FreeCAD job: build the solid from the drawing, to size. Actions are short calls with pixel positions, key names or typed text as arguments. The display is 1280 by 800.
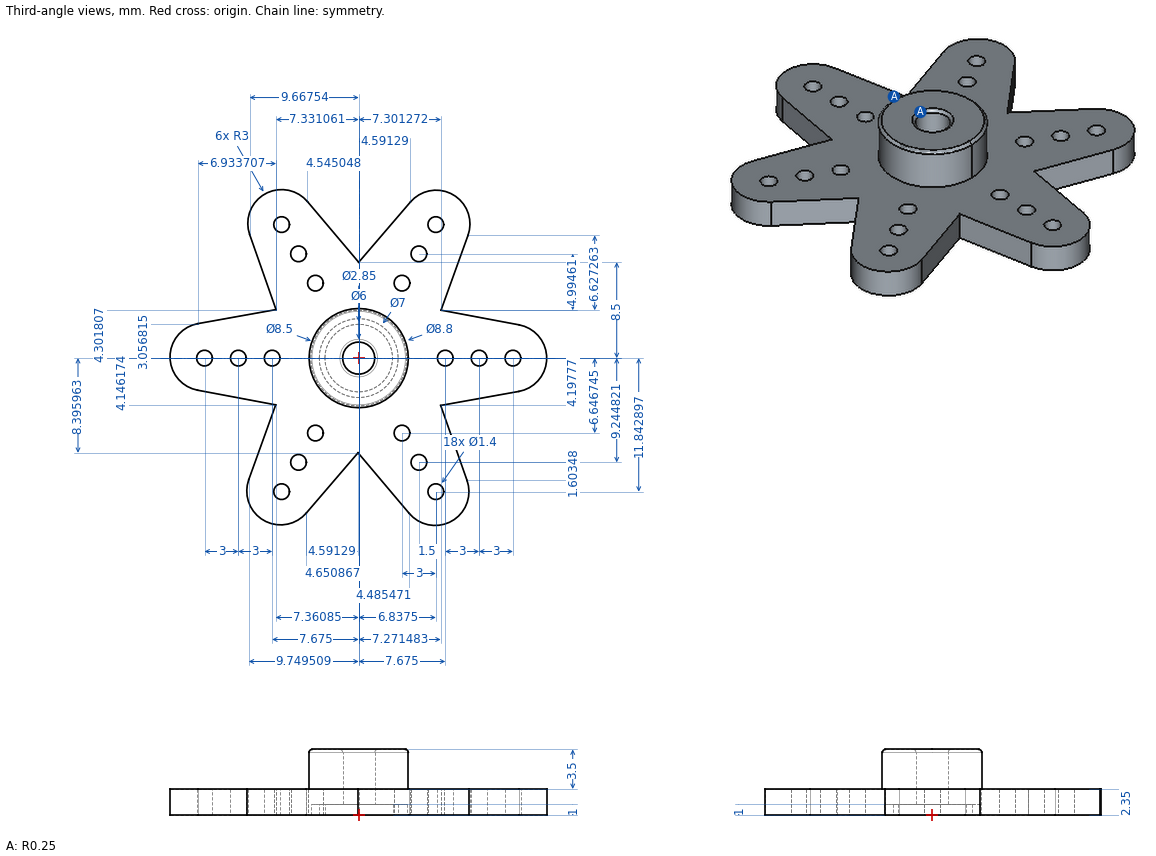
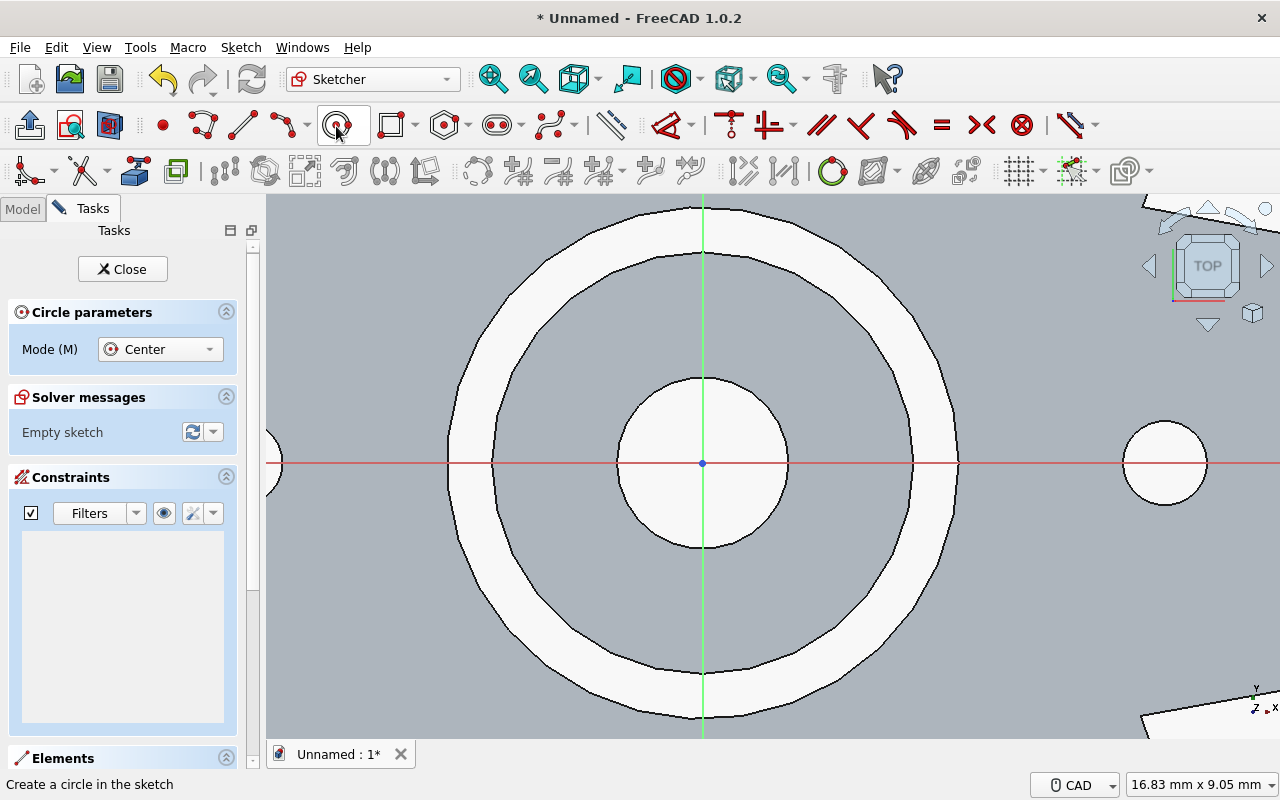
click(703, 463)
click(831, 335)
key(Escape)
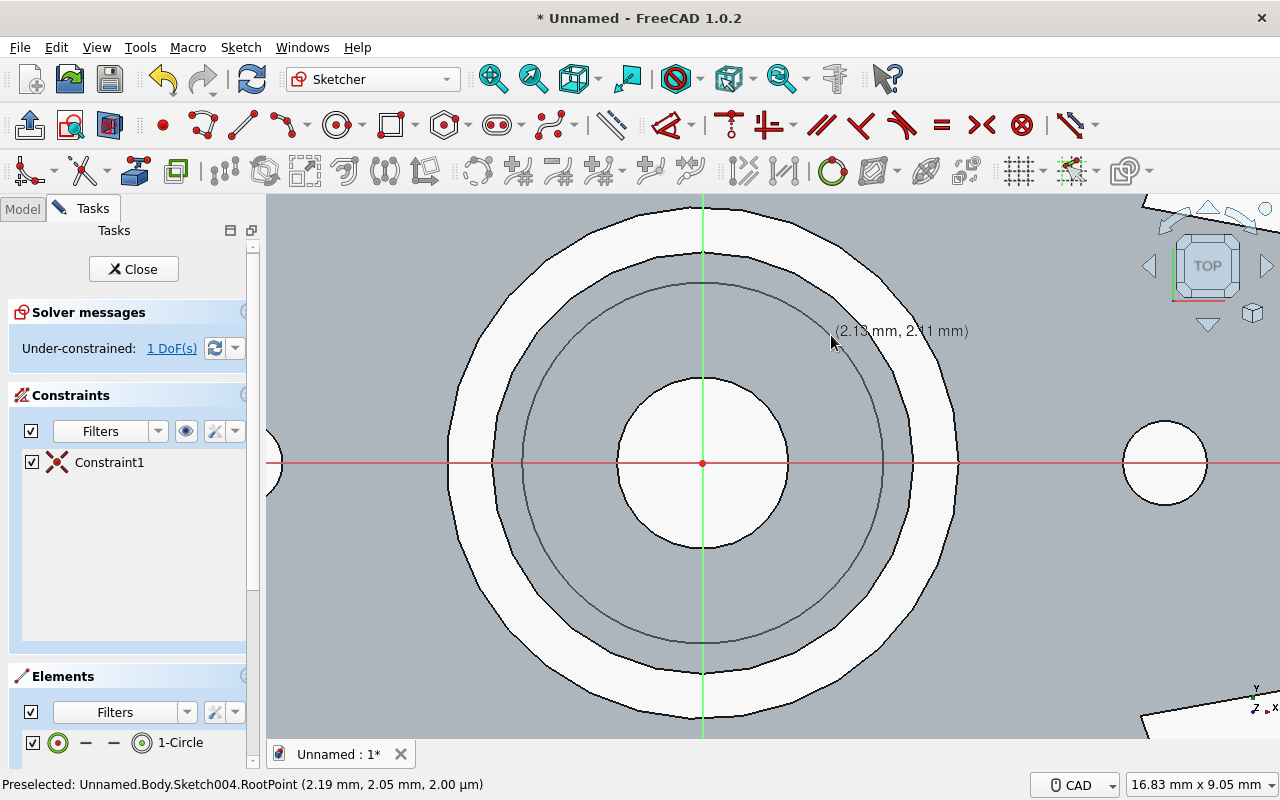
click(666, 126)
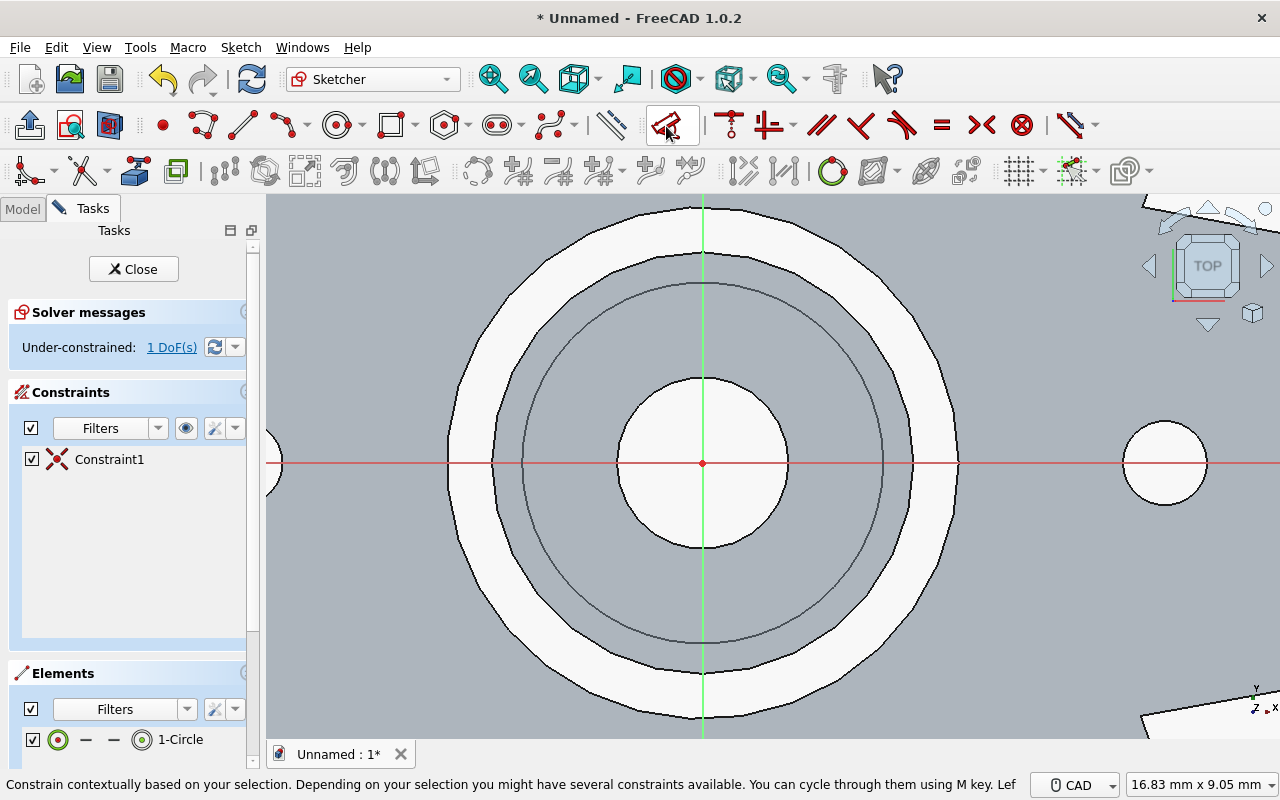
click(830, 335)
click(853, 312)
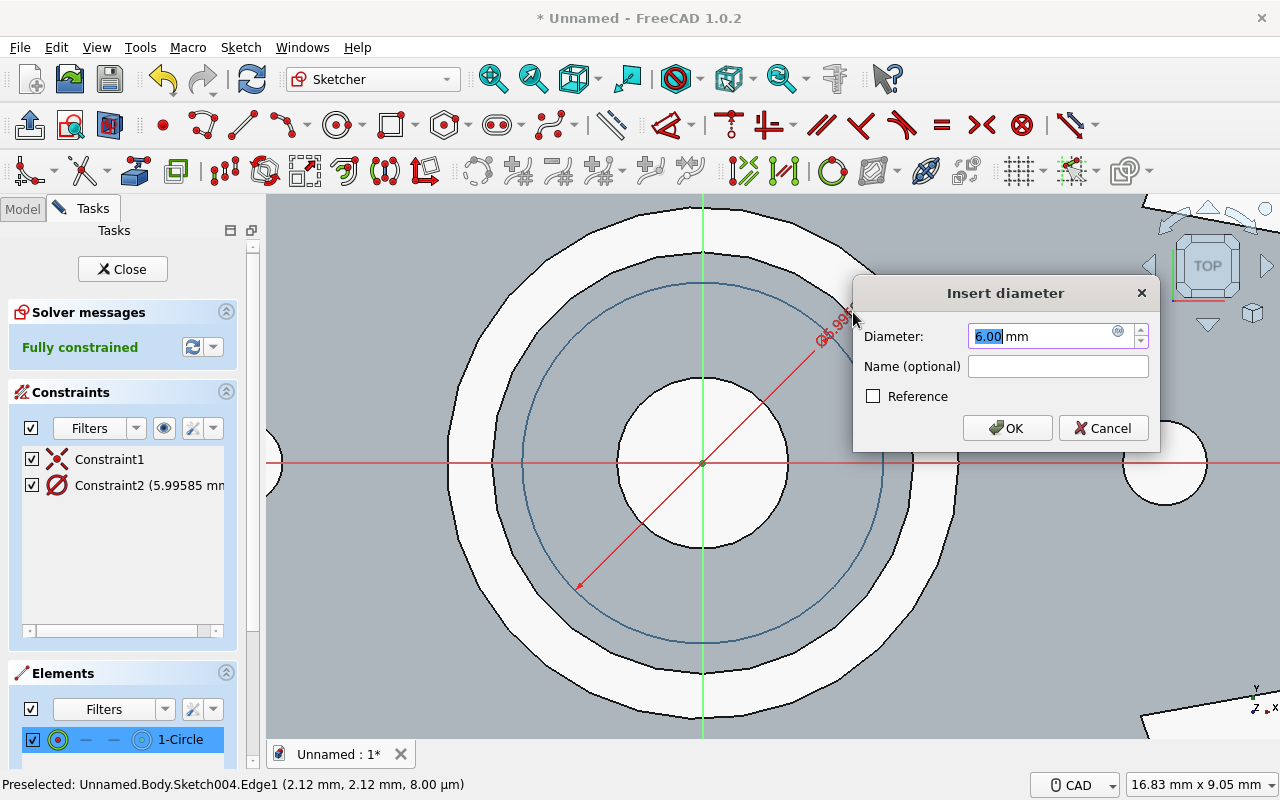
text(6)
key(Return)
key(Escape)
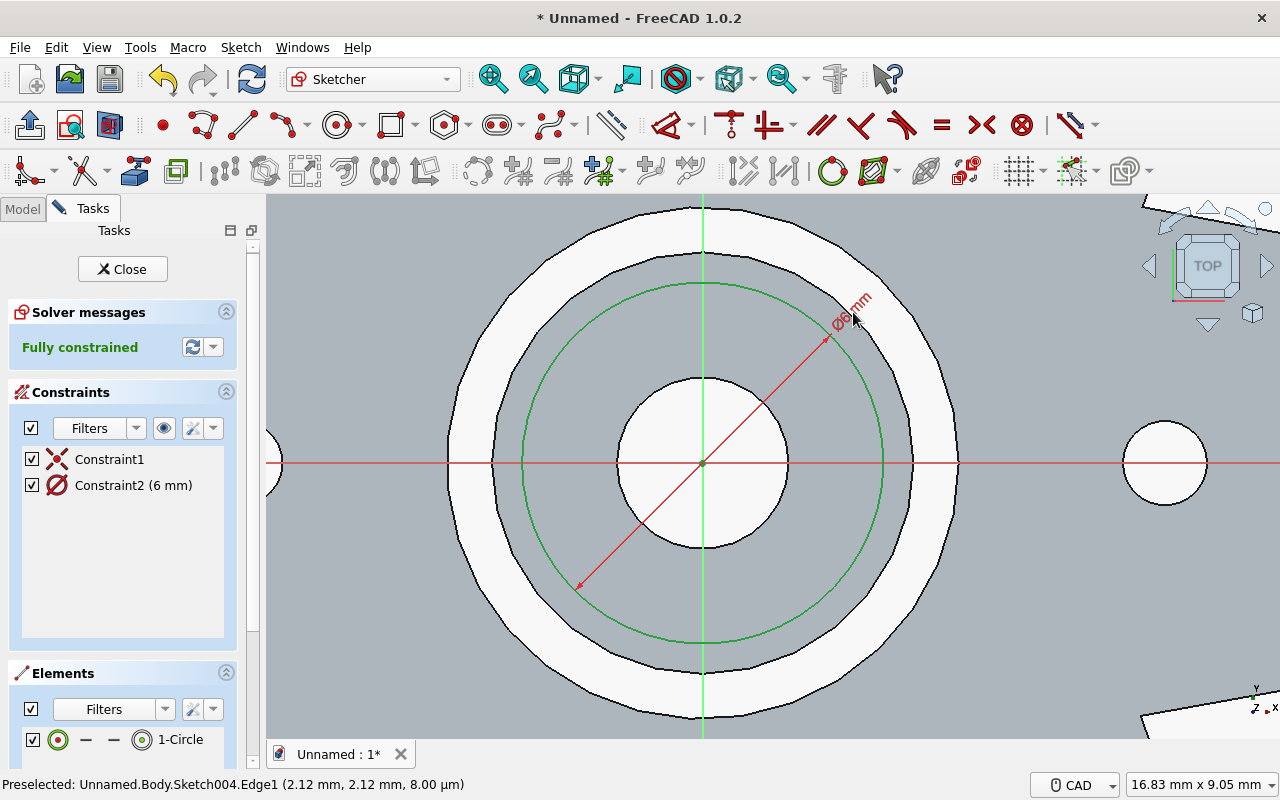
click(123, 269)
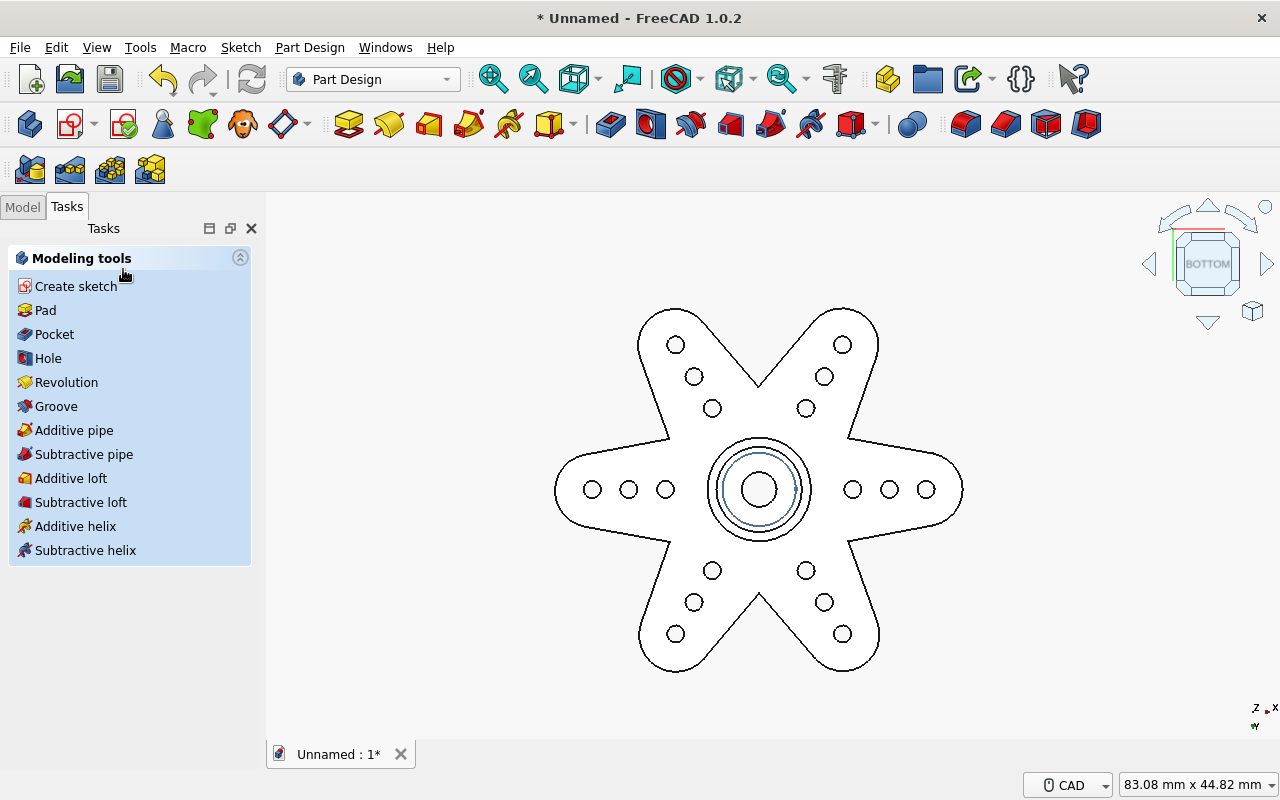
click(612, 124)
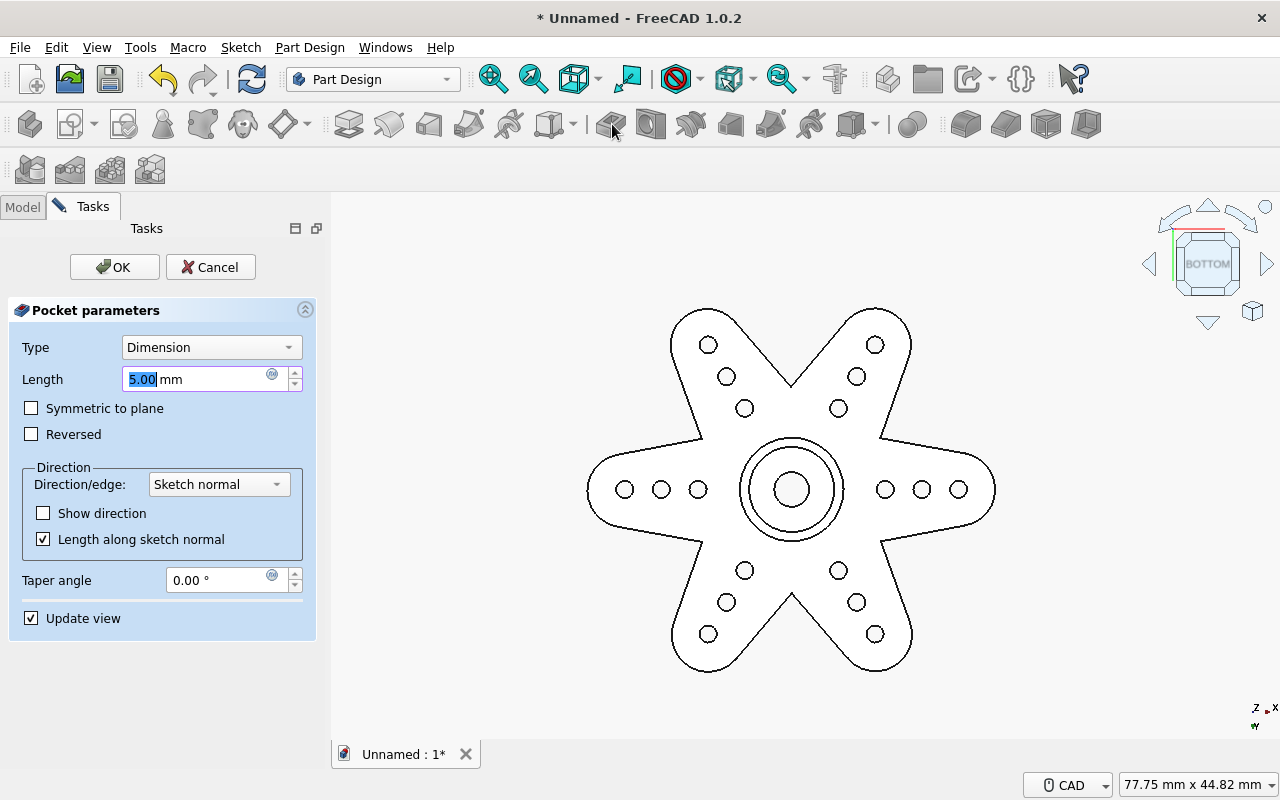
text(1)
key(Tab)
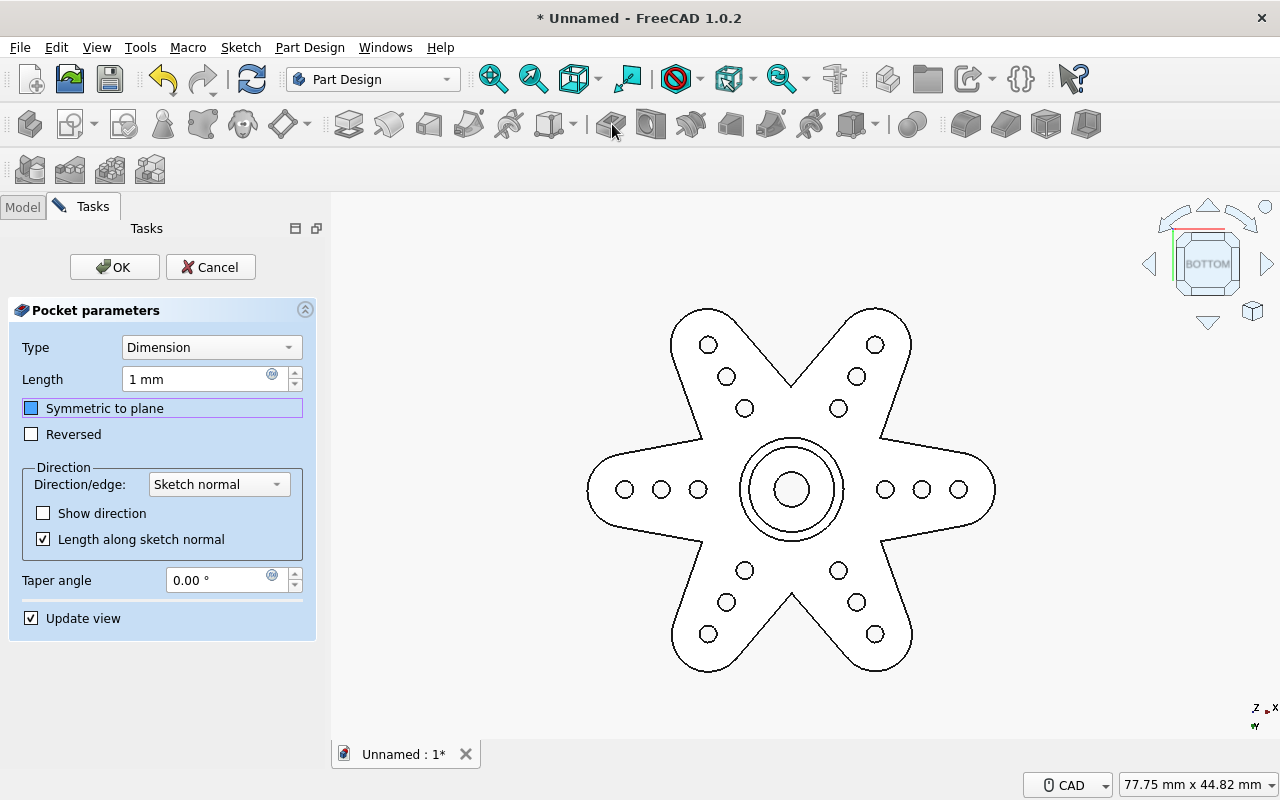
click(30, 434)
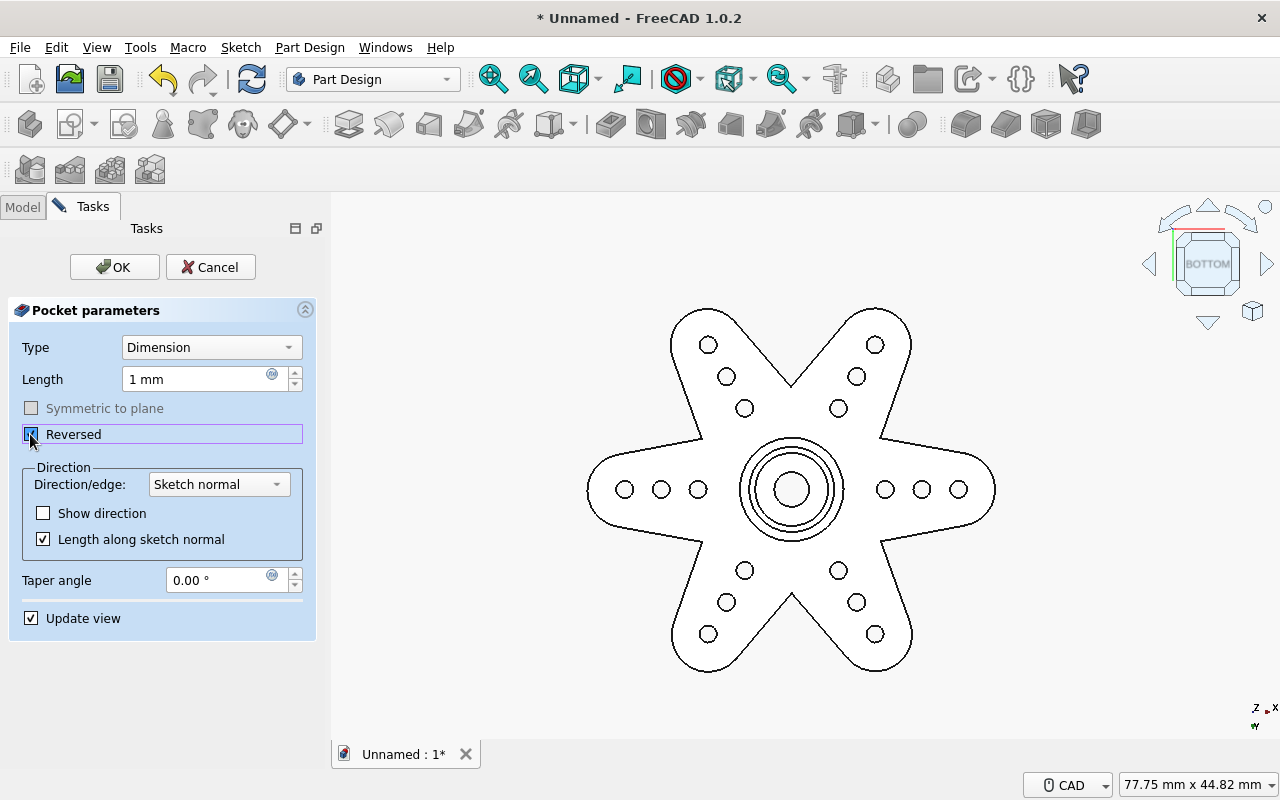
click(115, 267)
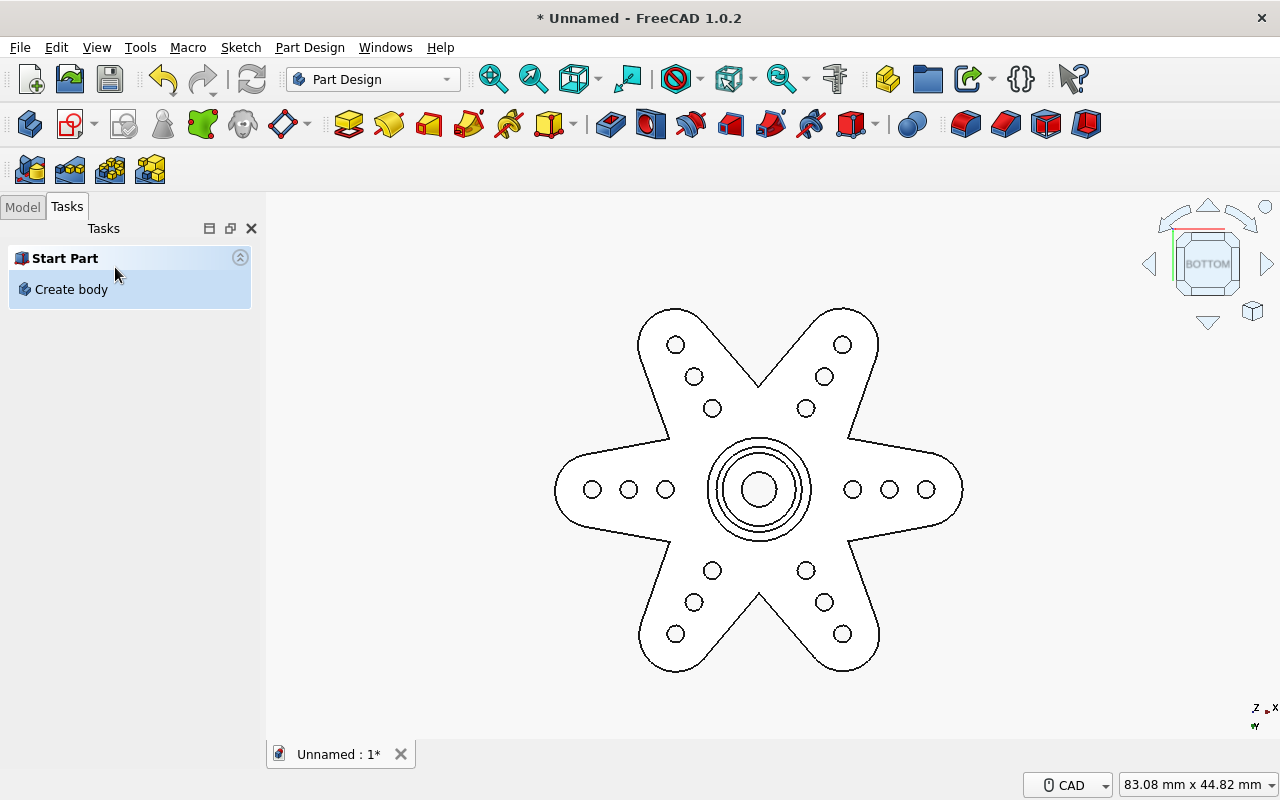
key(0)